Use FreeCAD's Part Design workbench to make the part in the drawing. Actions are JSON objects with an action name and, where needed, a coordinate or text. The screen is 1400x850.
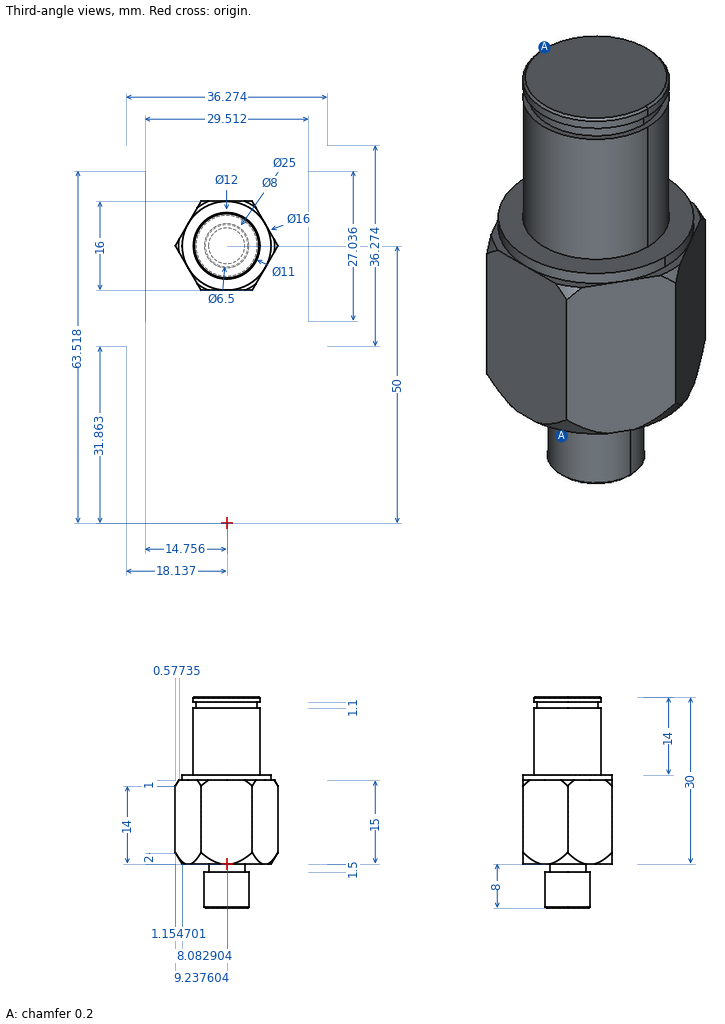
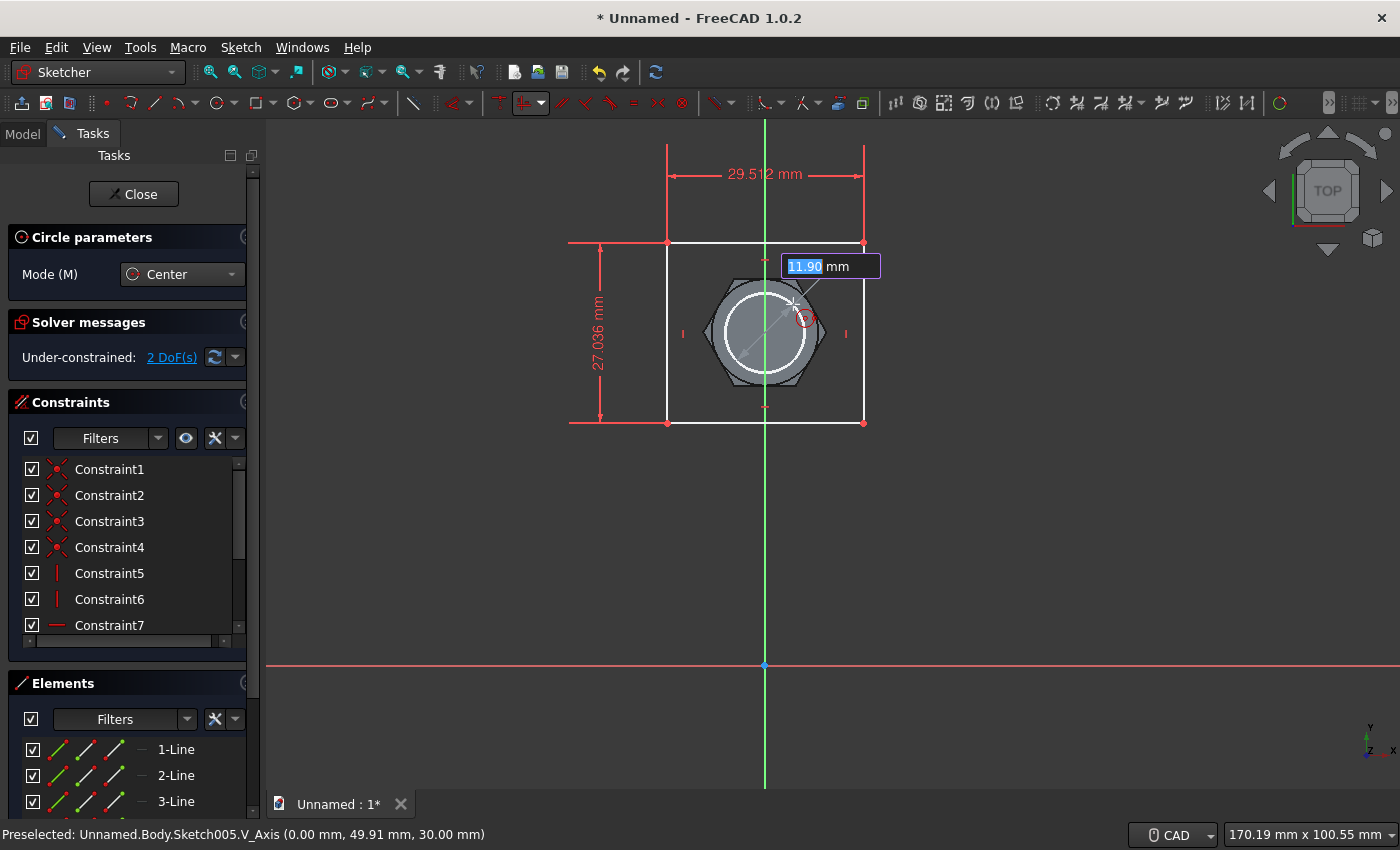
{"action": "type", "text": "12"}
{"action": "key", "text": "Return"}
{"action": "key", "text": "Escape"}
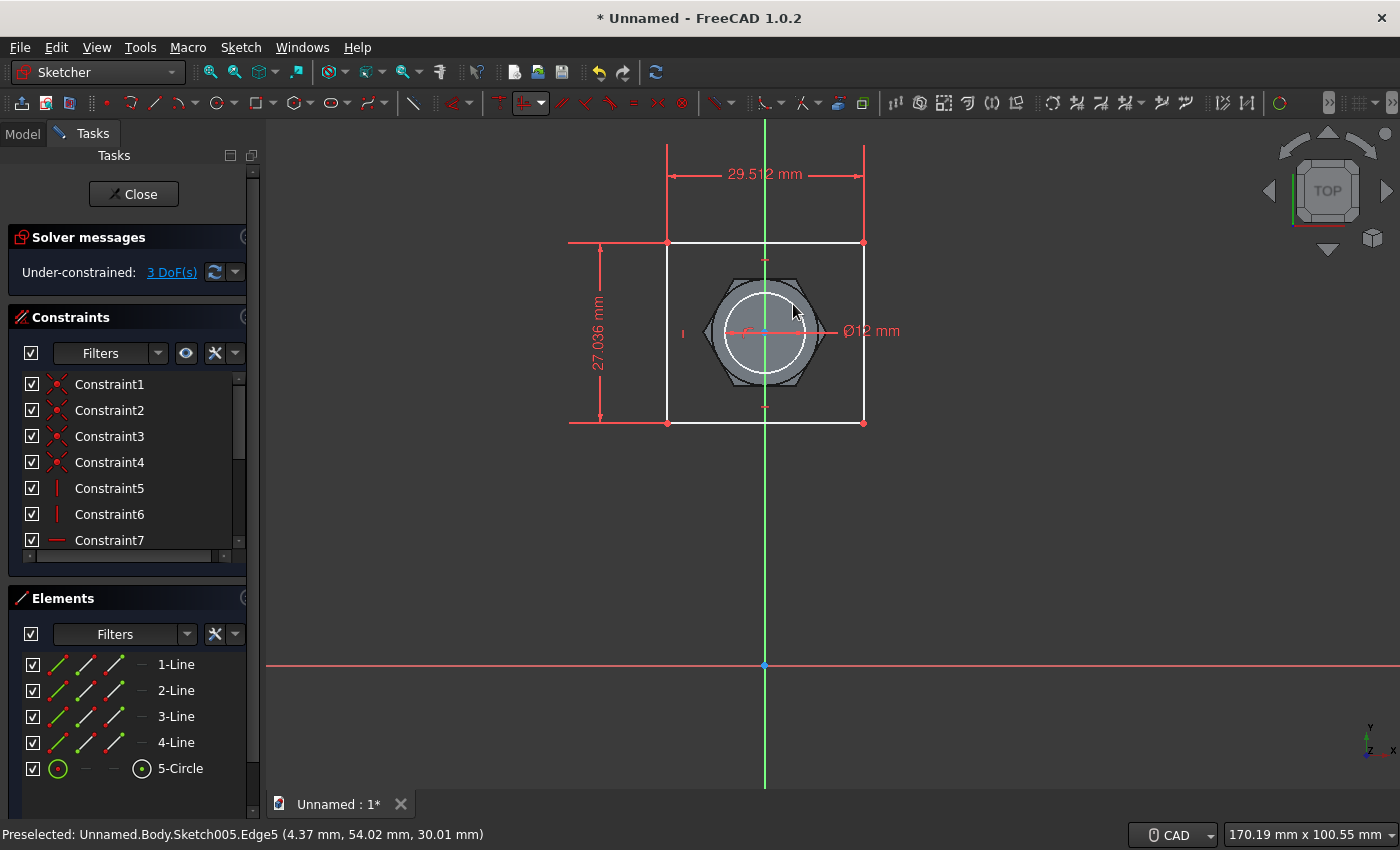
{"action": "left_click", "coordinate": [452, 104]}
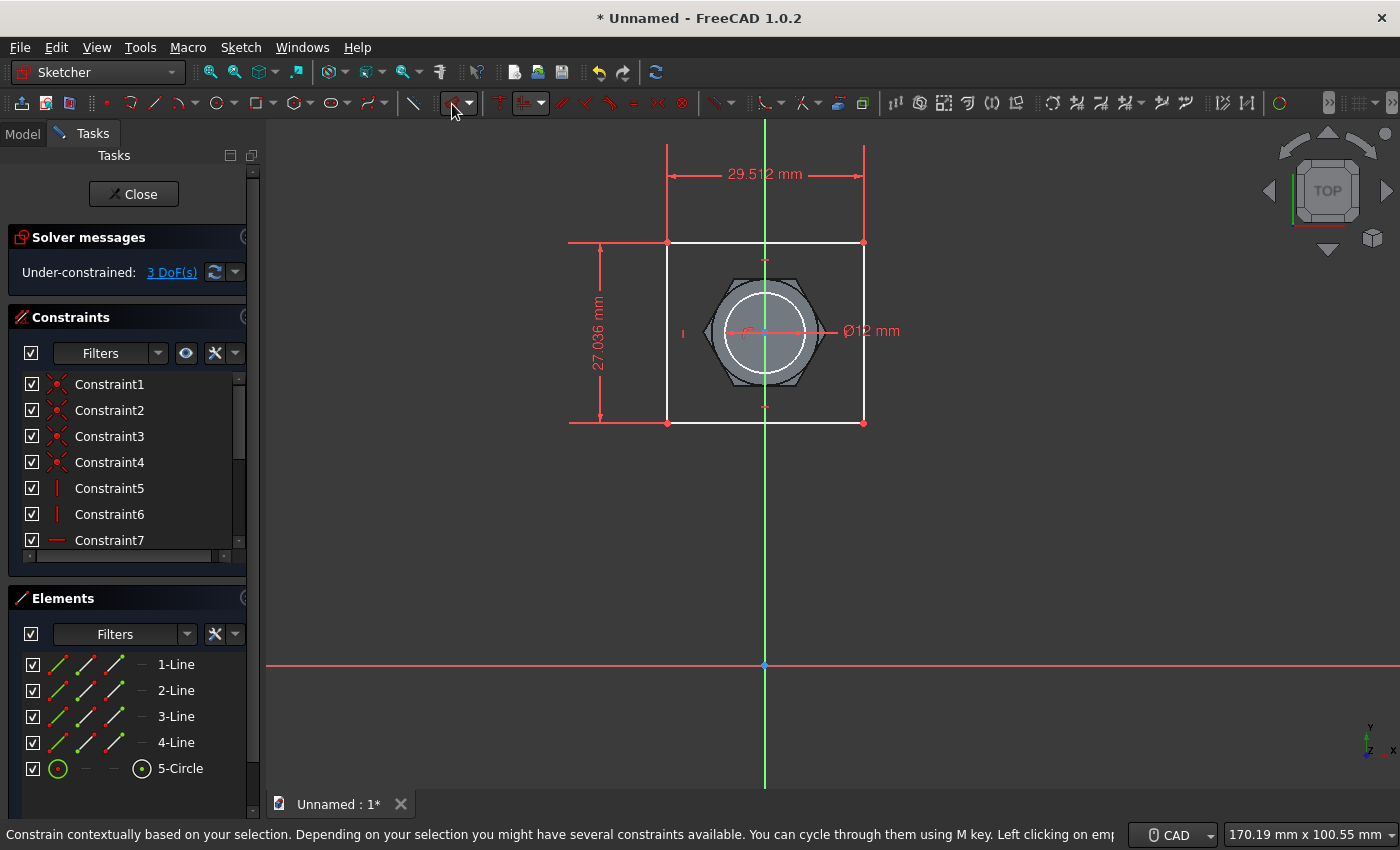
{"action": "left_click", "coordinate": [765, 333]}
{"action": "left_click", "coordinate": [799, 499]}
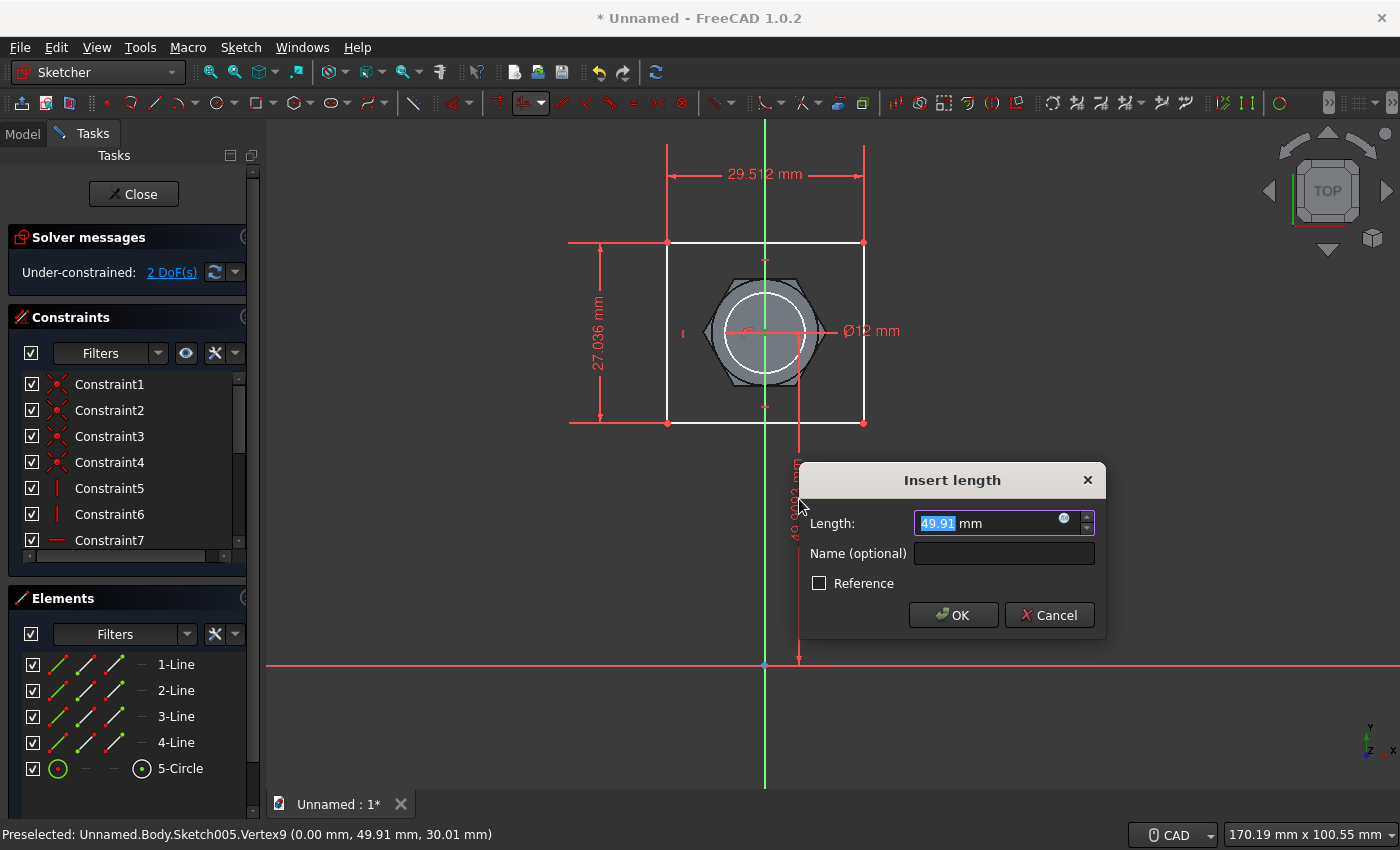
{"action": "type", "text": "50"}
{"action": "key", "text": "Return"}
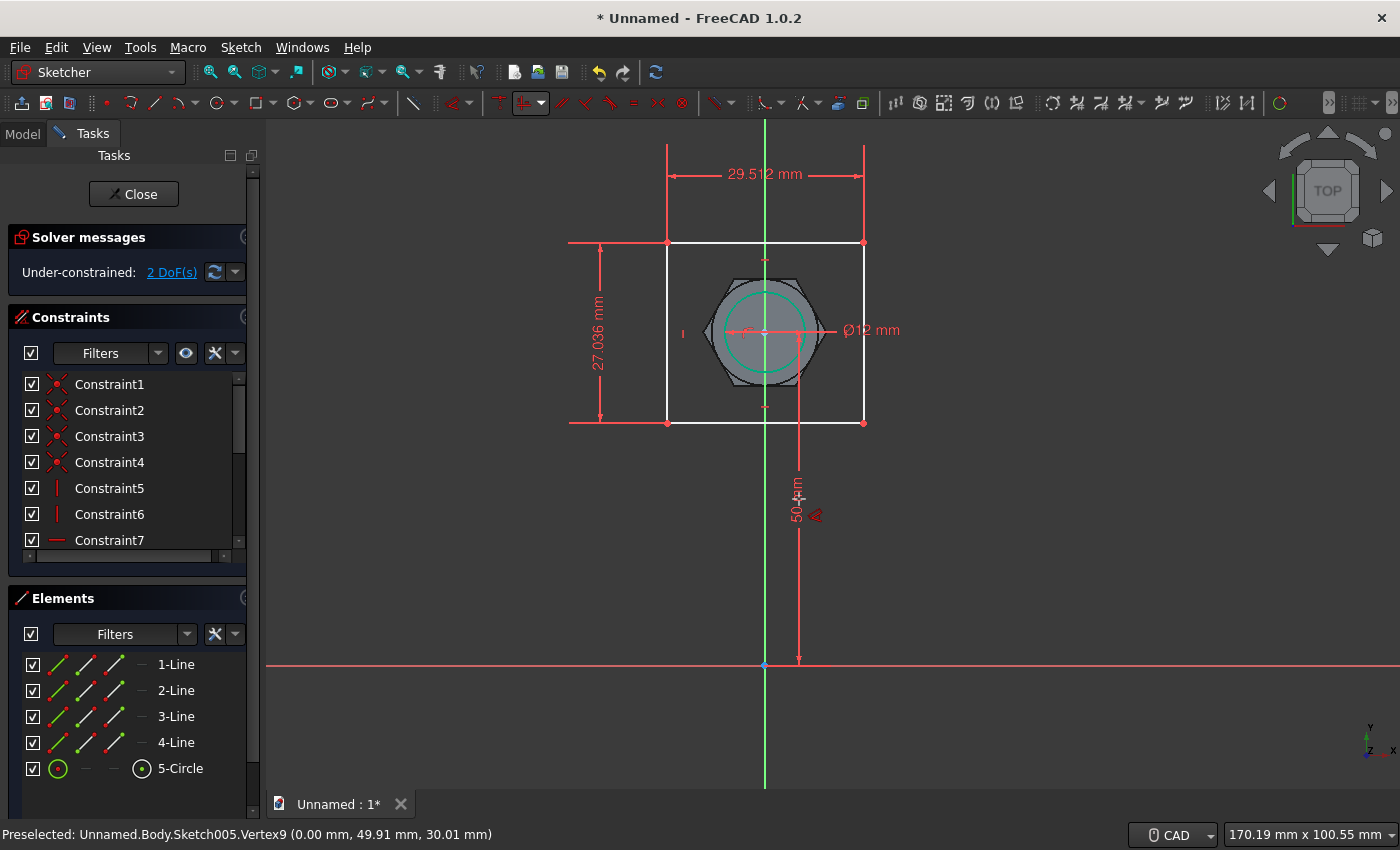
{"action": "left_click", "coordinate": [667, 243]}
{"action": "left_click", "coordinate": [716, 700]}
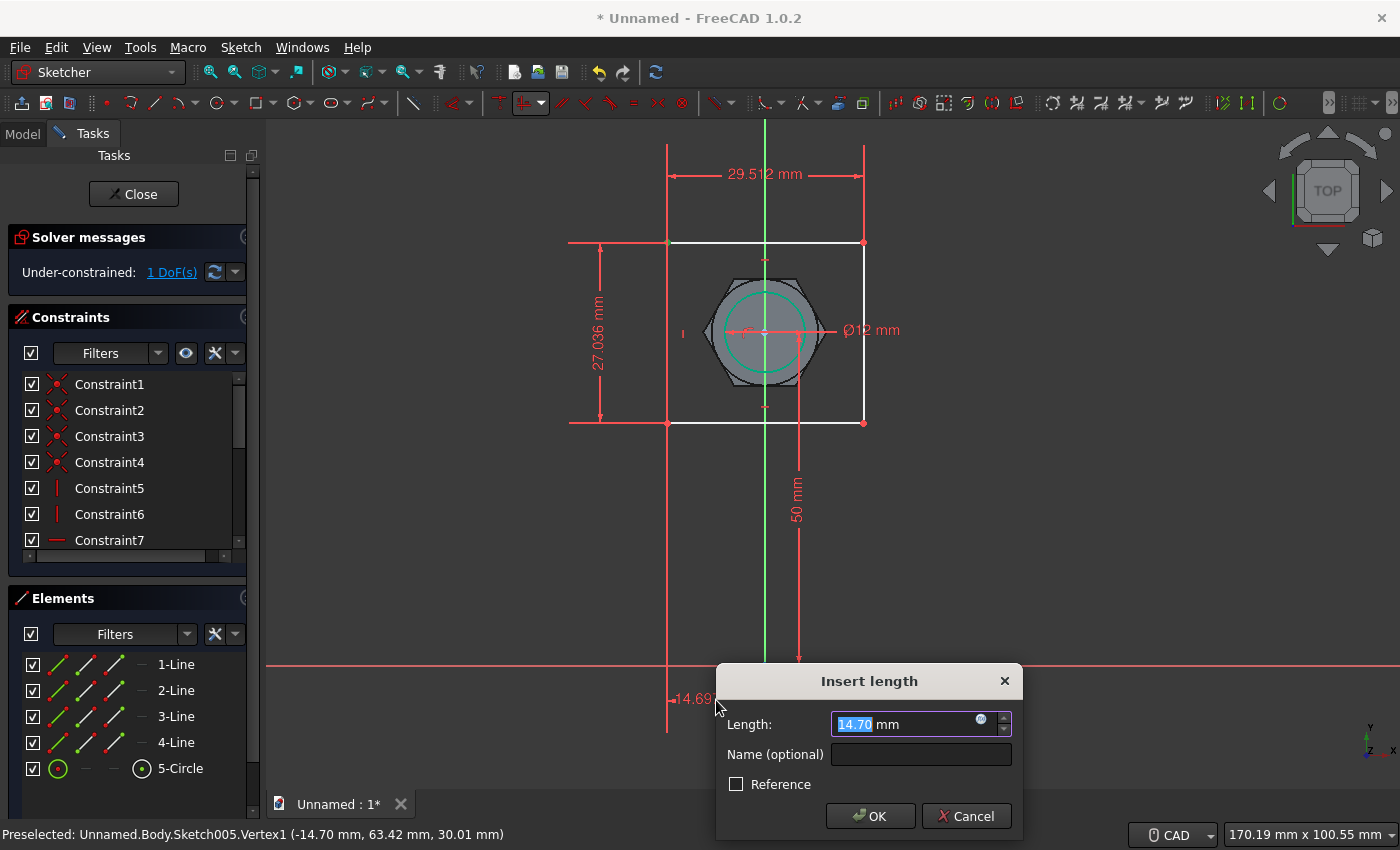
{"action": "type", "text": "14.756"}
{"action": "key", "text": "Return"}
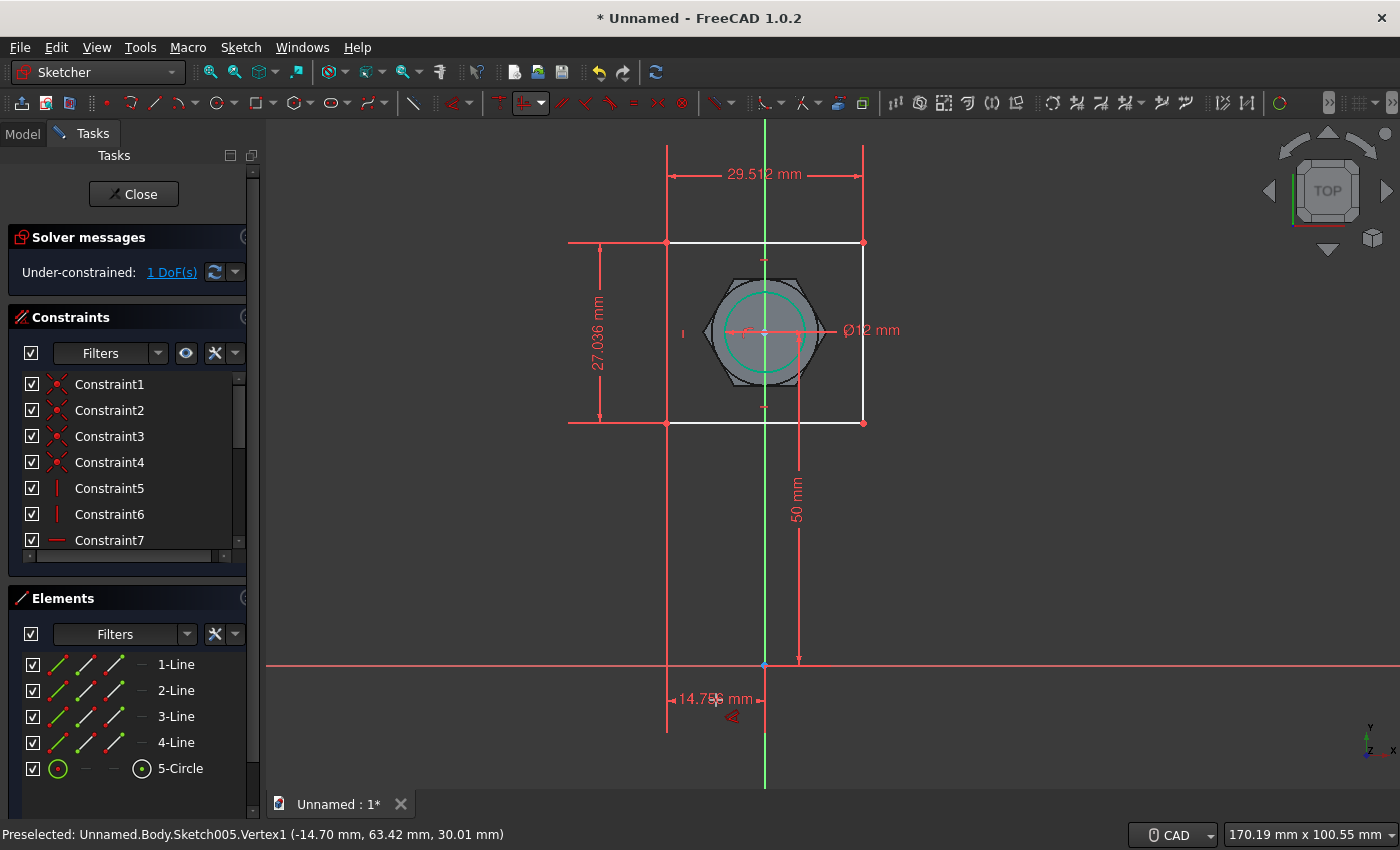
{"action": "left_click", "coordinate": [667, 243]}
{"action": "left_click", "coordinate": [633, 454]}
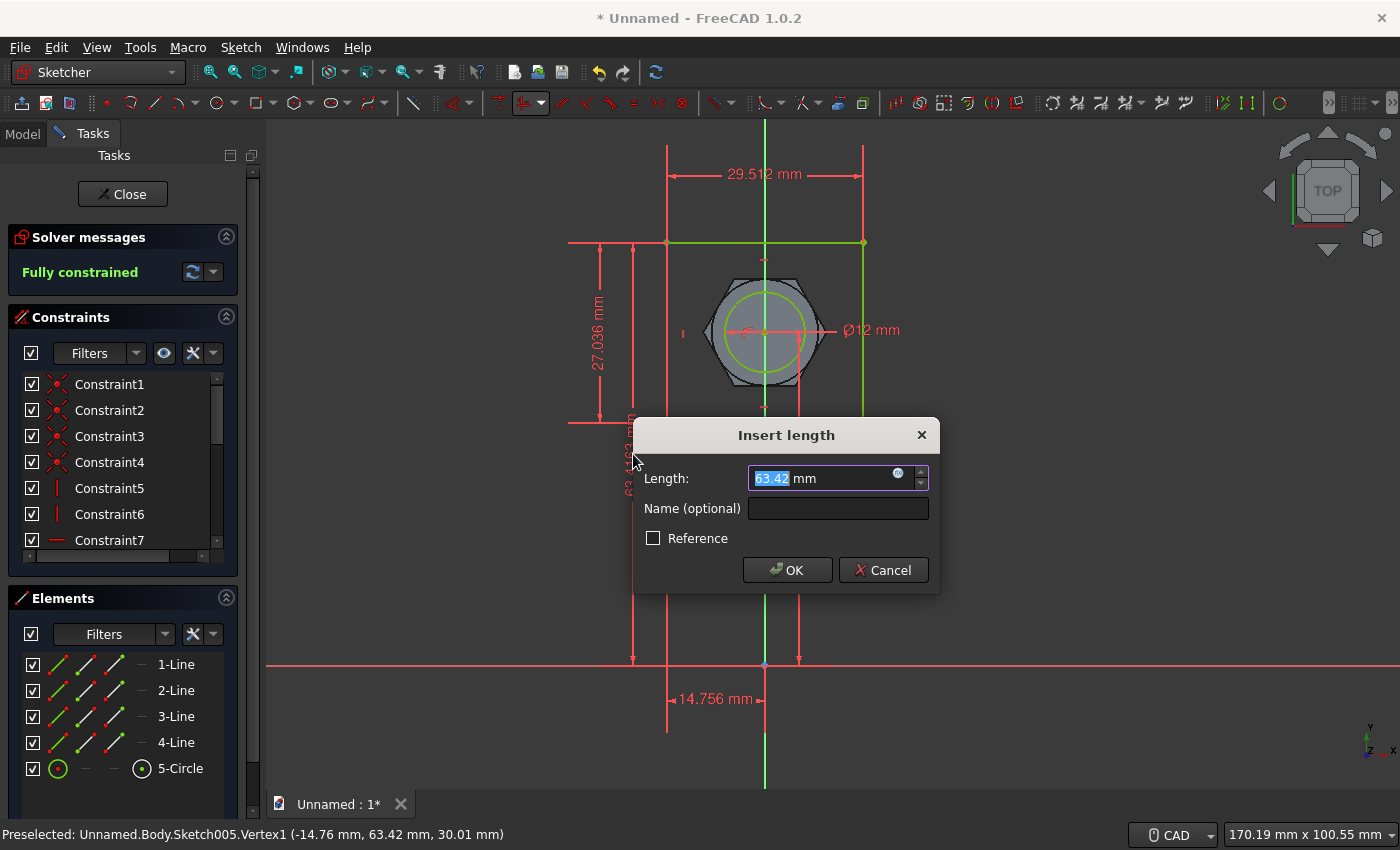
{"action": "type", "text": "63.518"}
{"action": "key", "text": "Return"}
{"action": "key", "text": "Escape"}